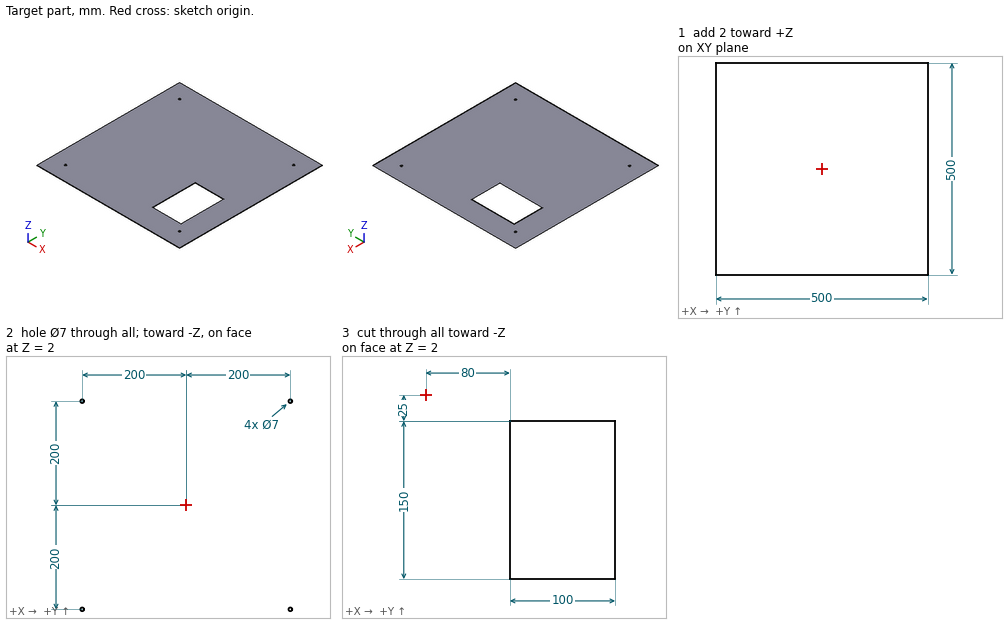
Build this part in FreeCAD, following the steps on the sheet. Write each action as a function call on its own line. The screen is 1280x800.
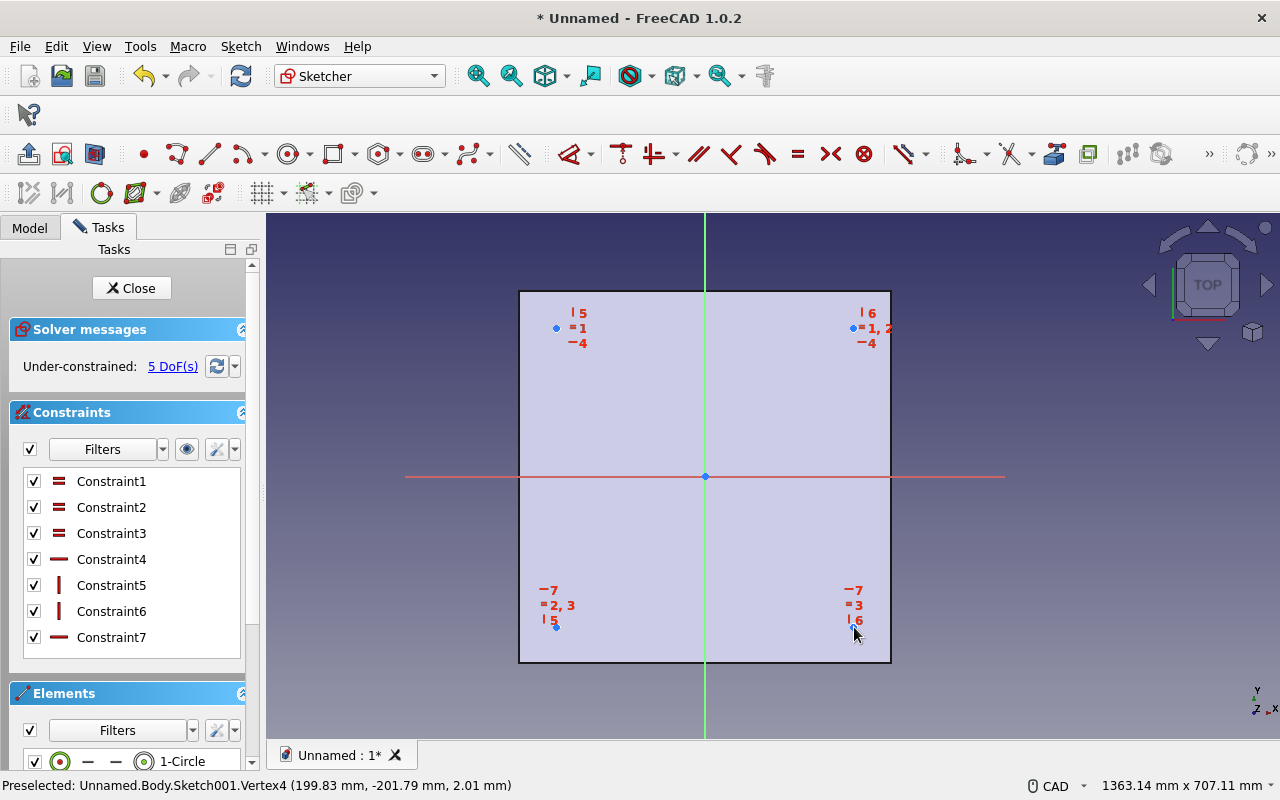
scroll(559, 327, up, 11)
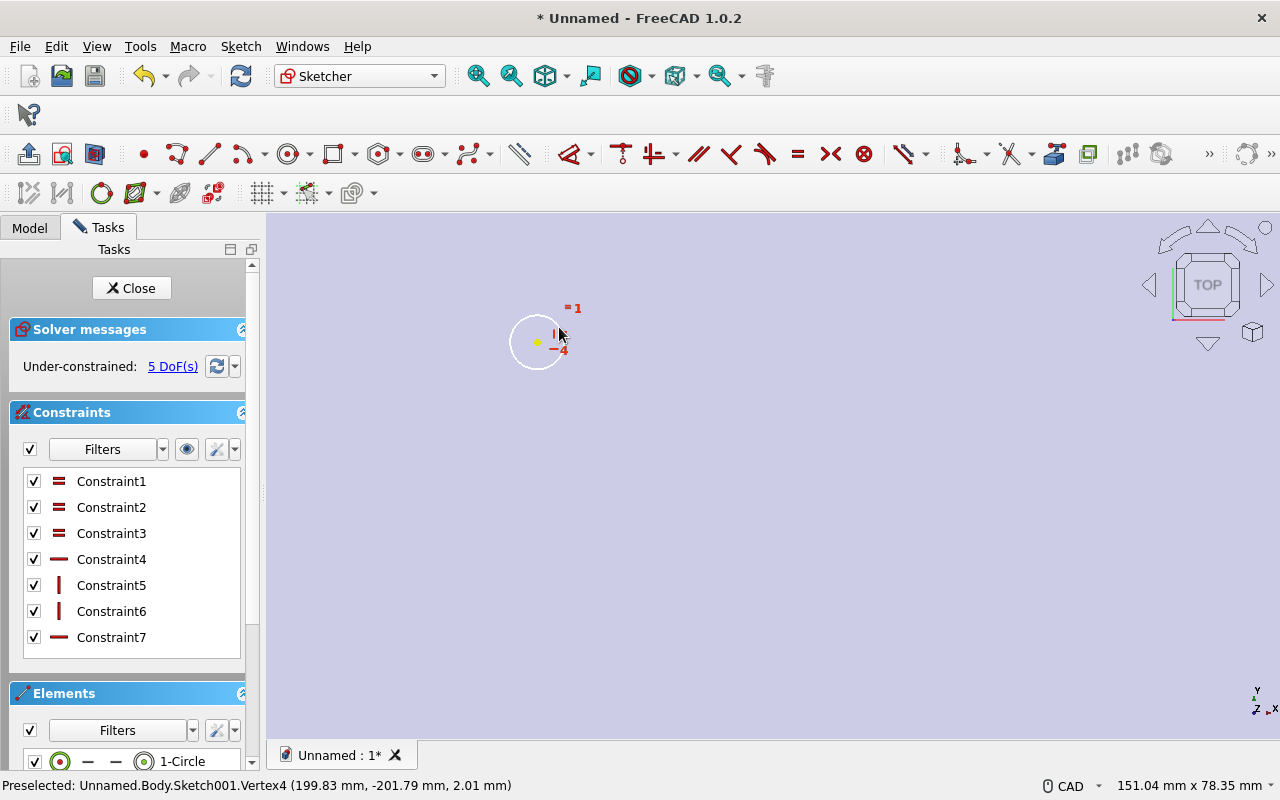
click(556, 323)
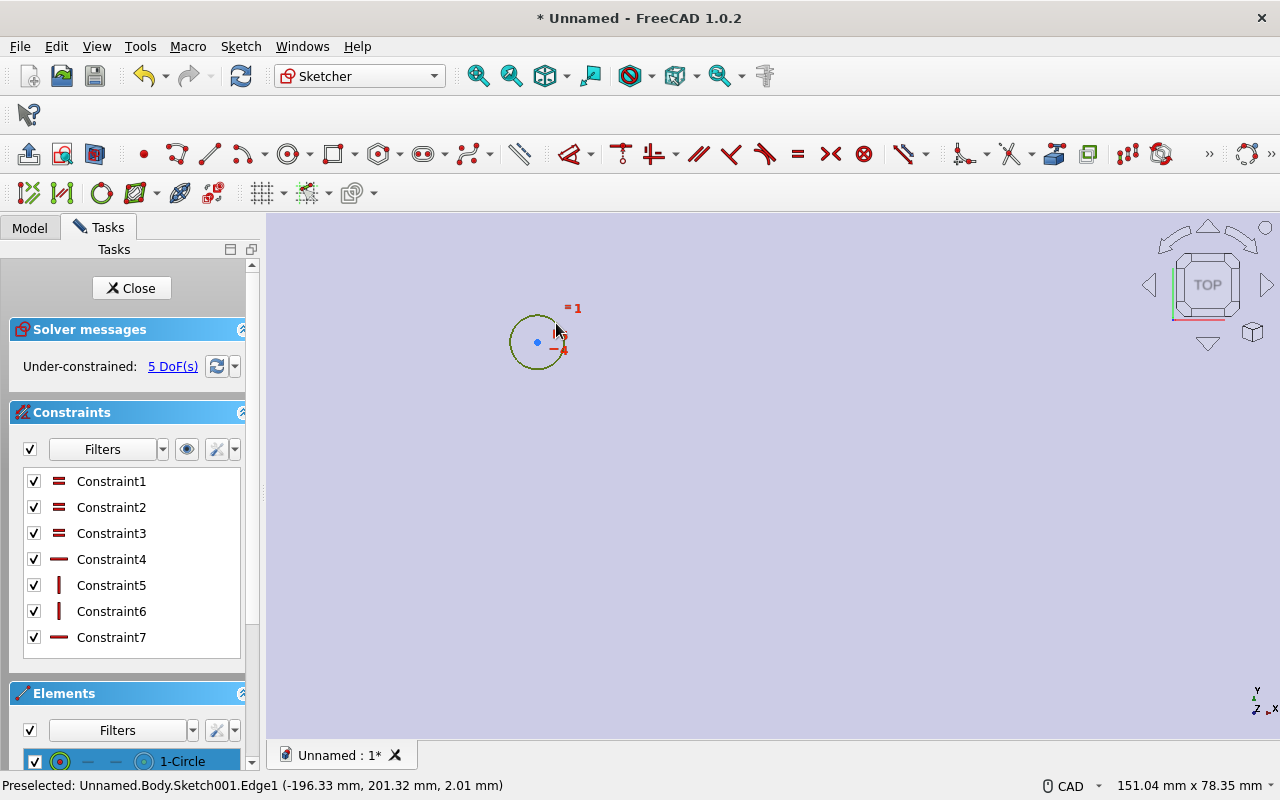
key(k)
key(o)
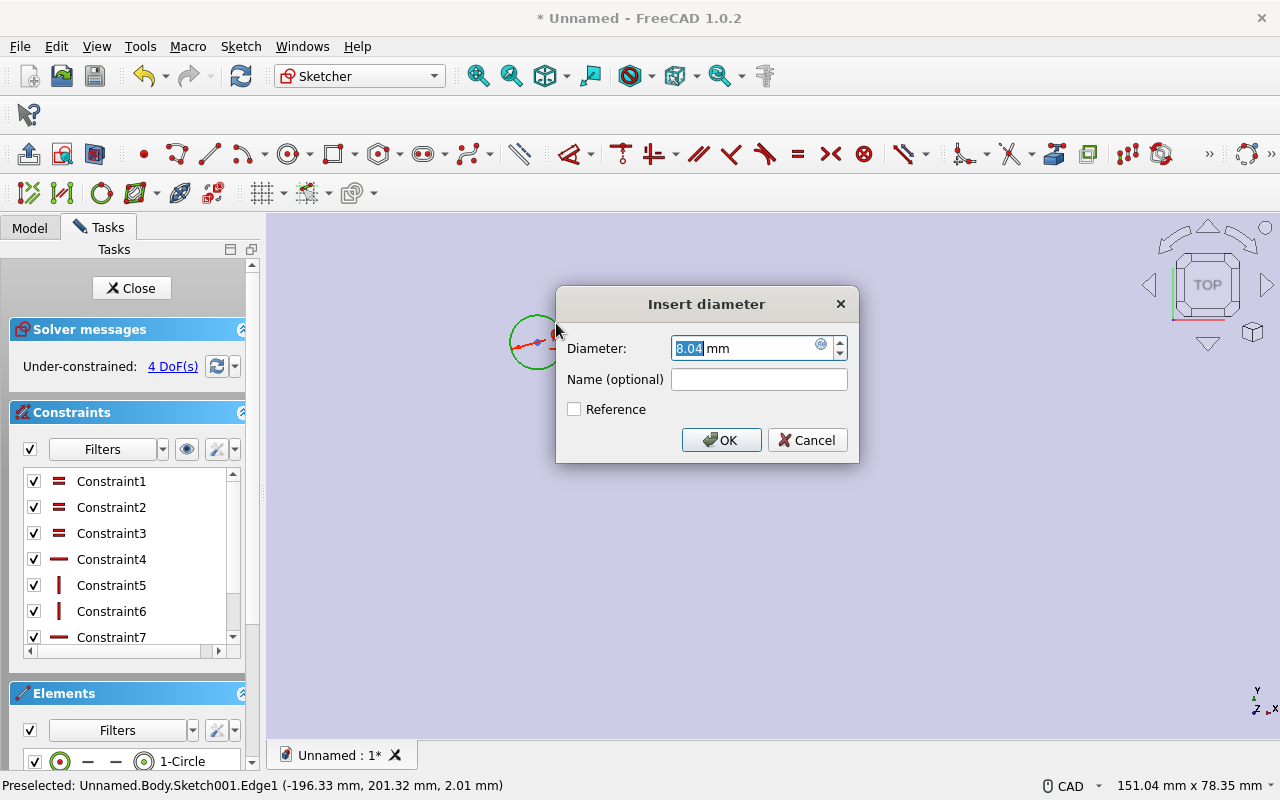
text(7)
key(Return)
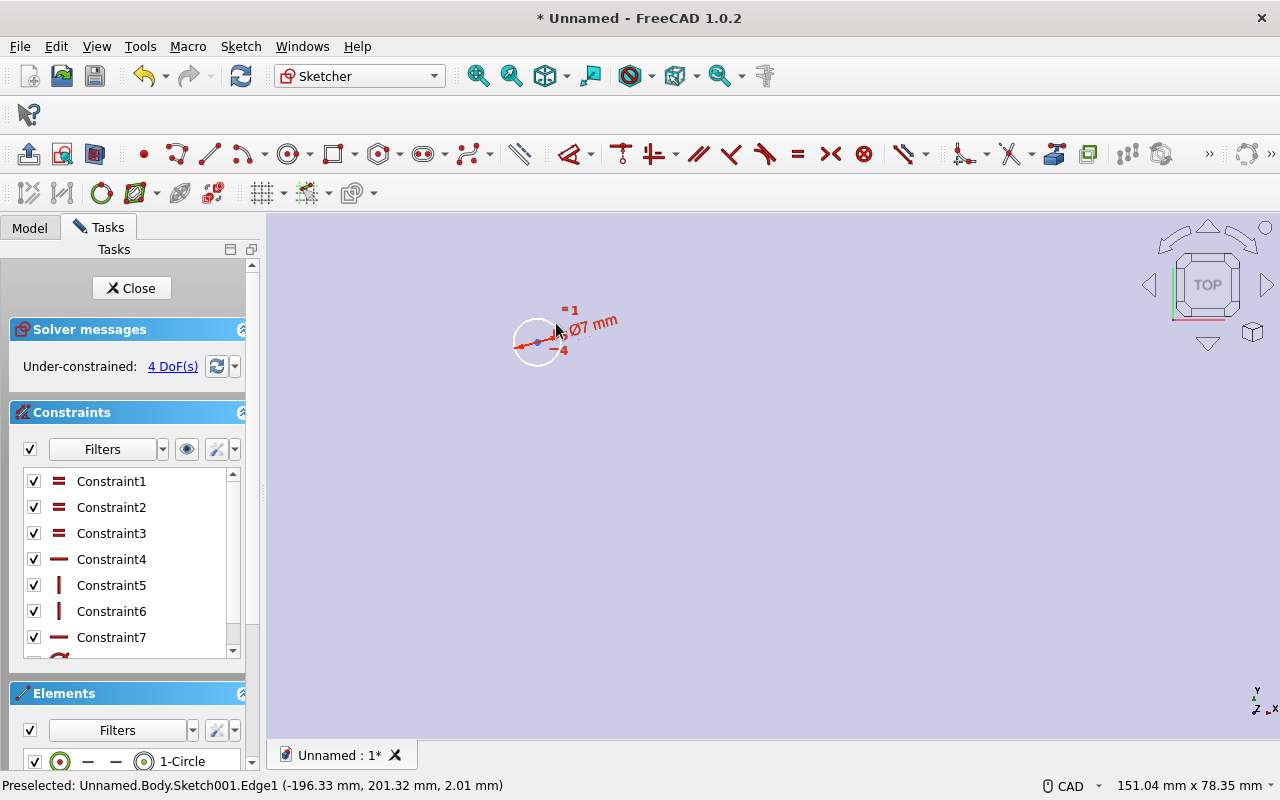
scroll(558, 326, down, 11)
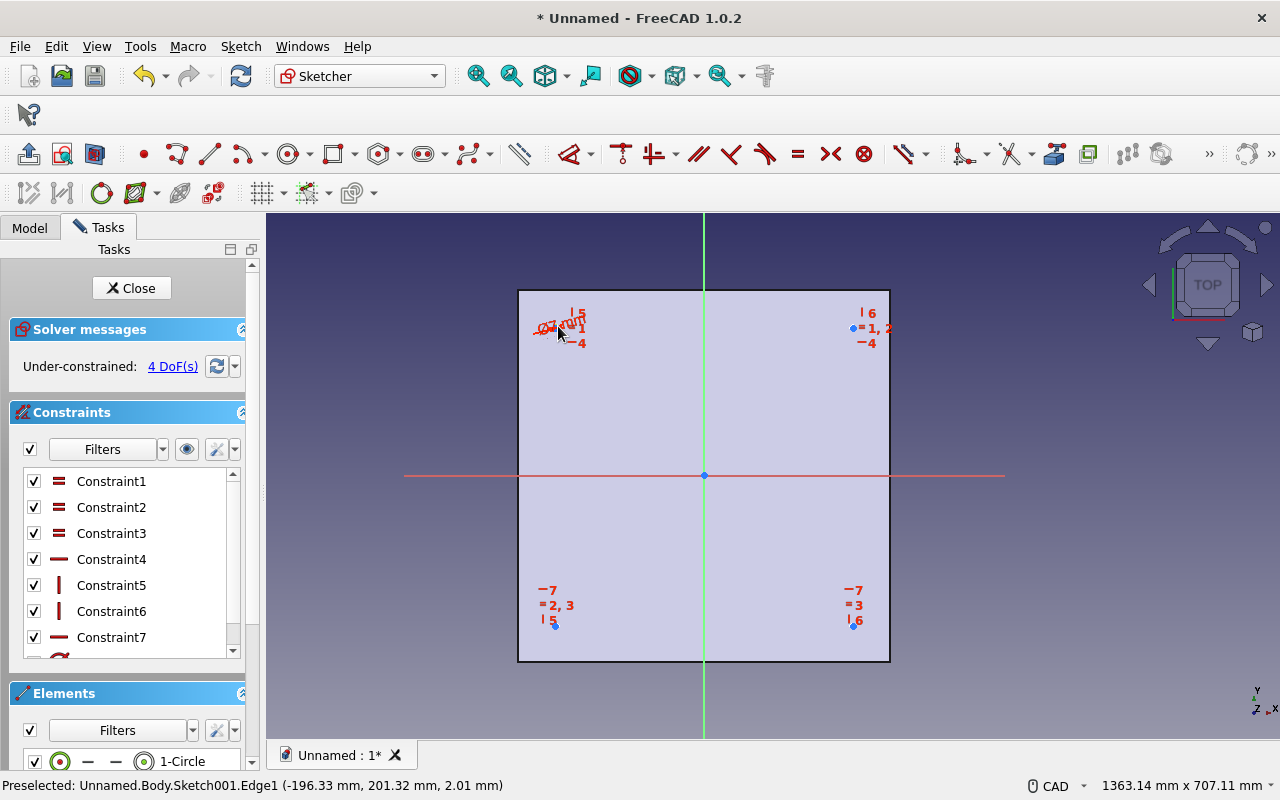
click(556, 328)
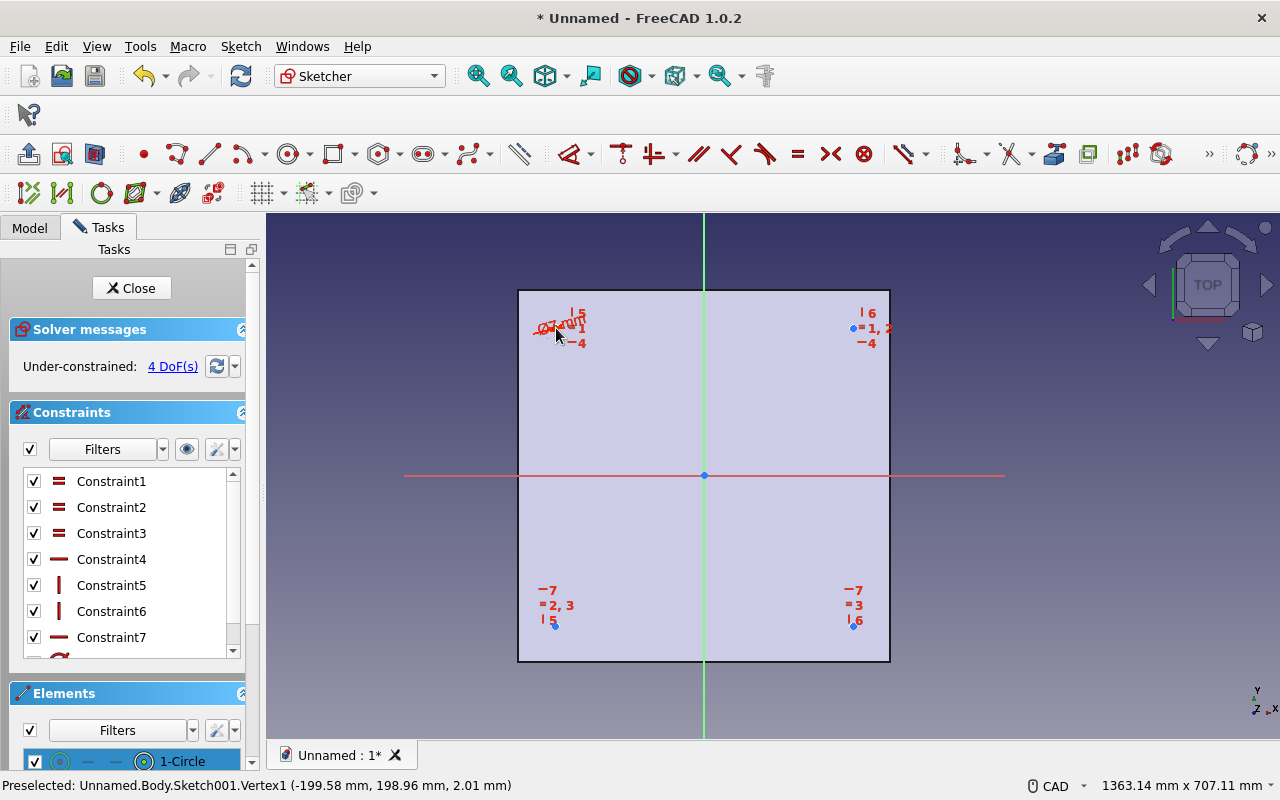
click(590, 154)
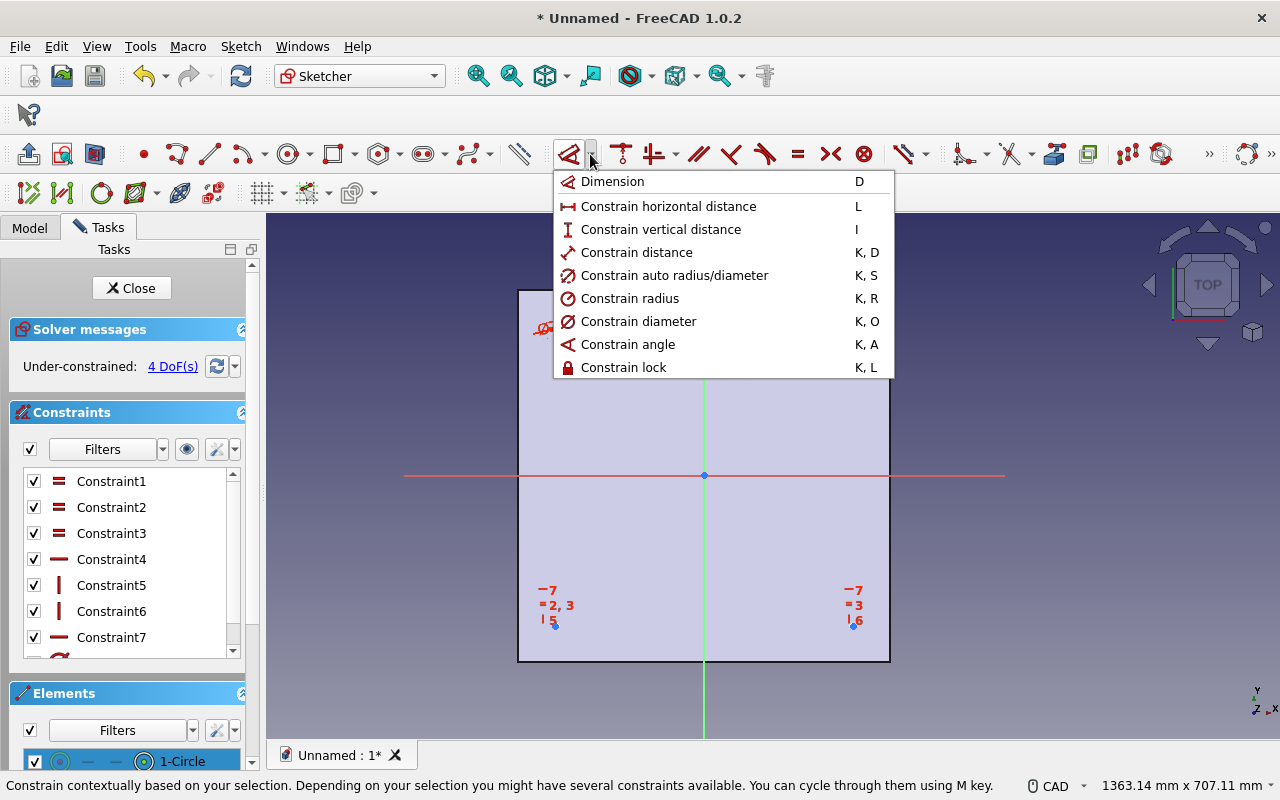
click(724, 206)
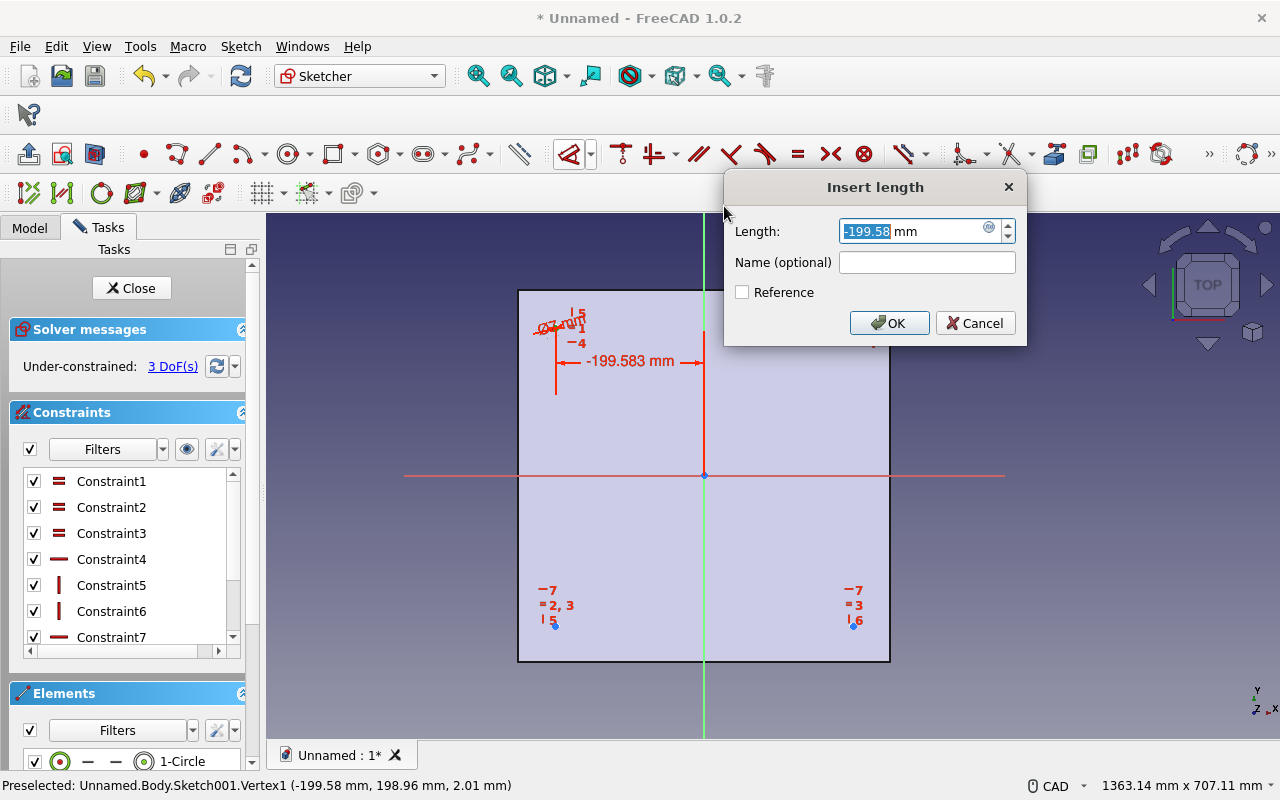
text(-200)
key(Return)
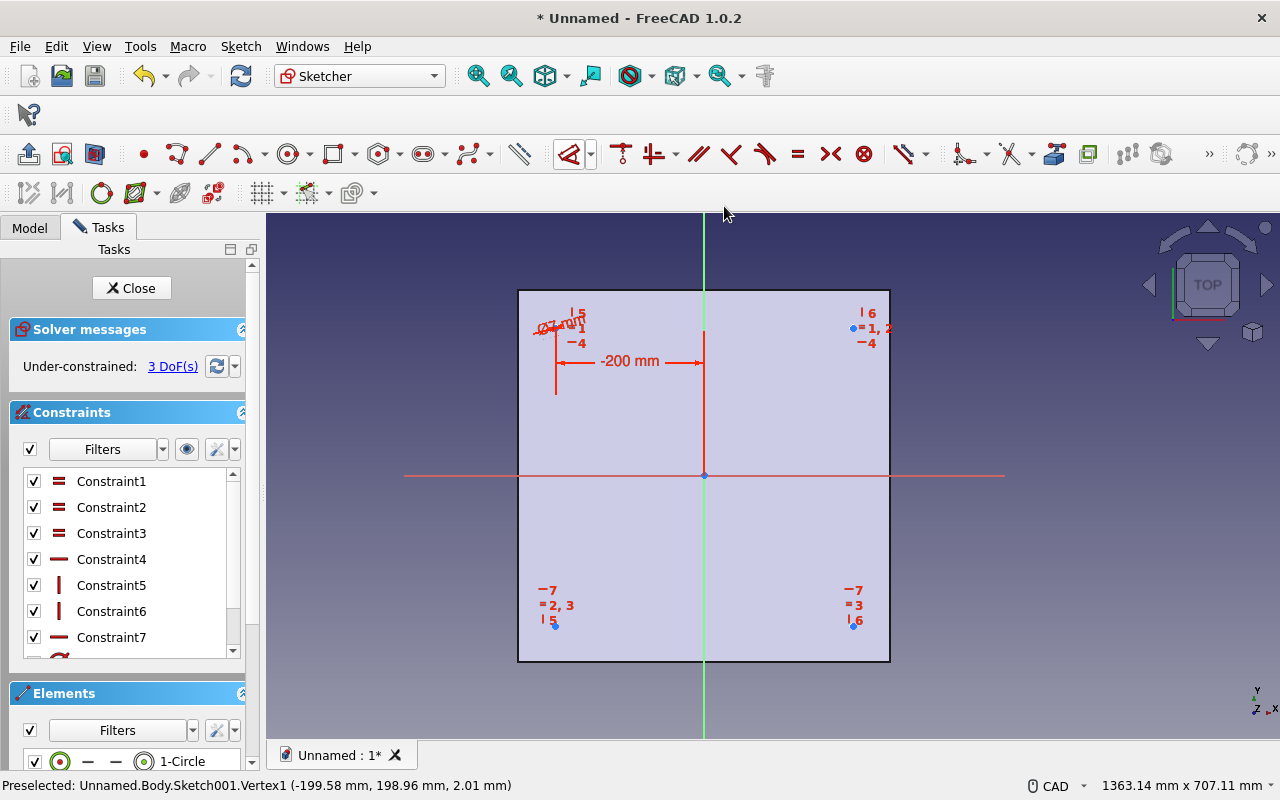
click(556, 328)